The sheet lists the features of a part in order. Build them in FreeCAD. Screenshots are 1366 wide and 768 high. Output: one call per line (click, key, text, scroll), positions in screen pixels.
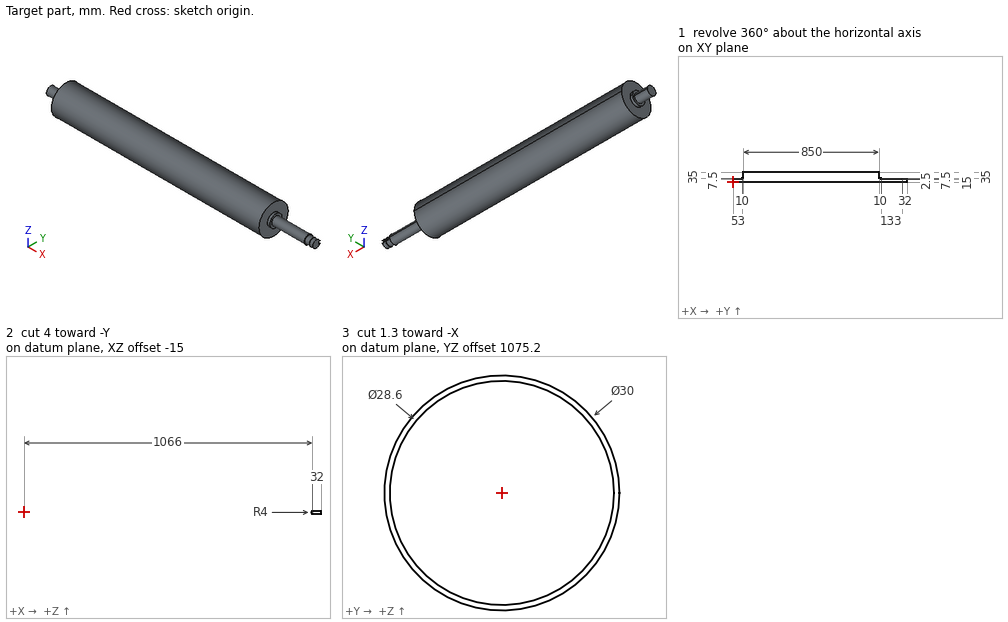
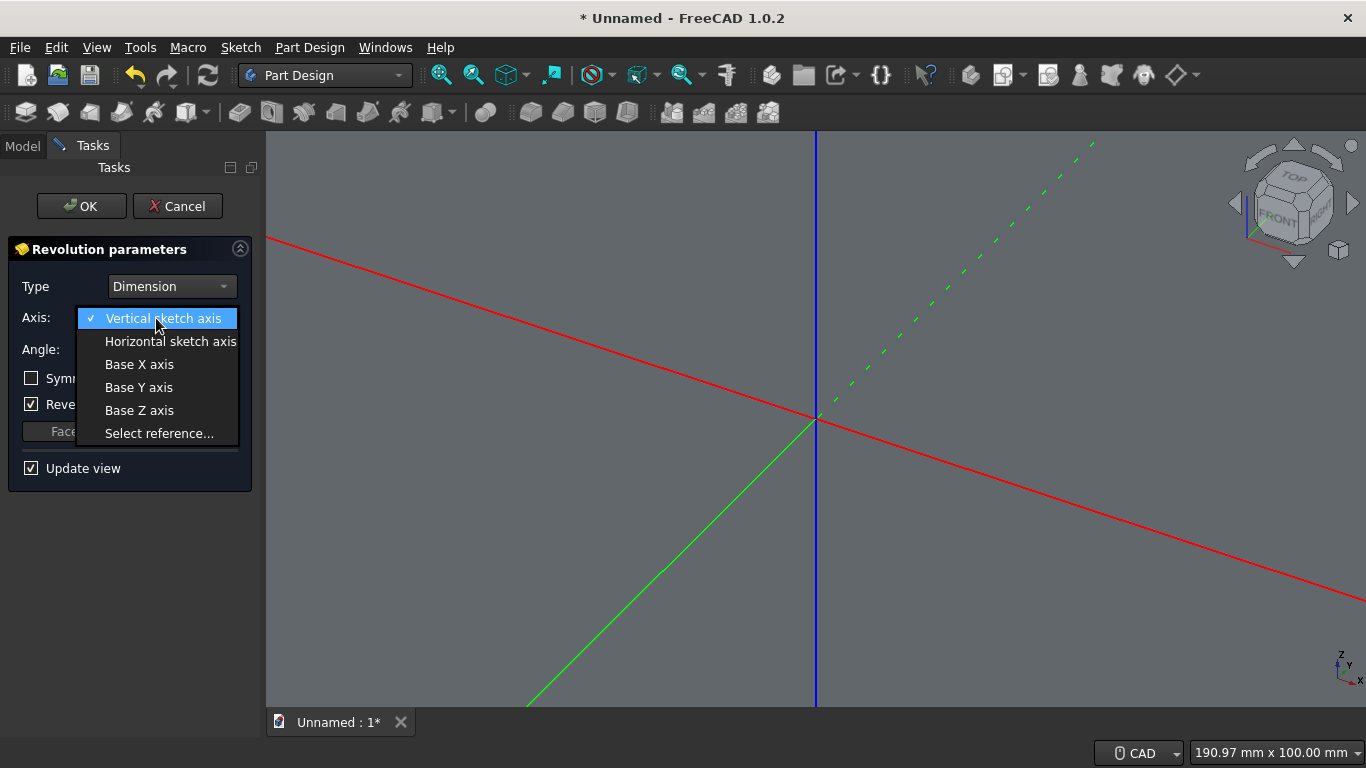
click(156, 342)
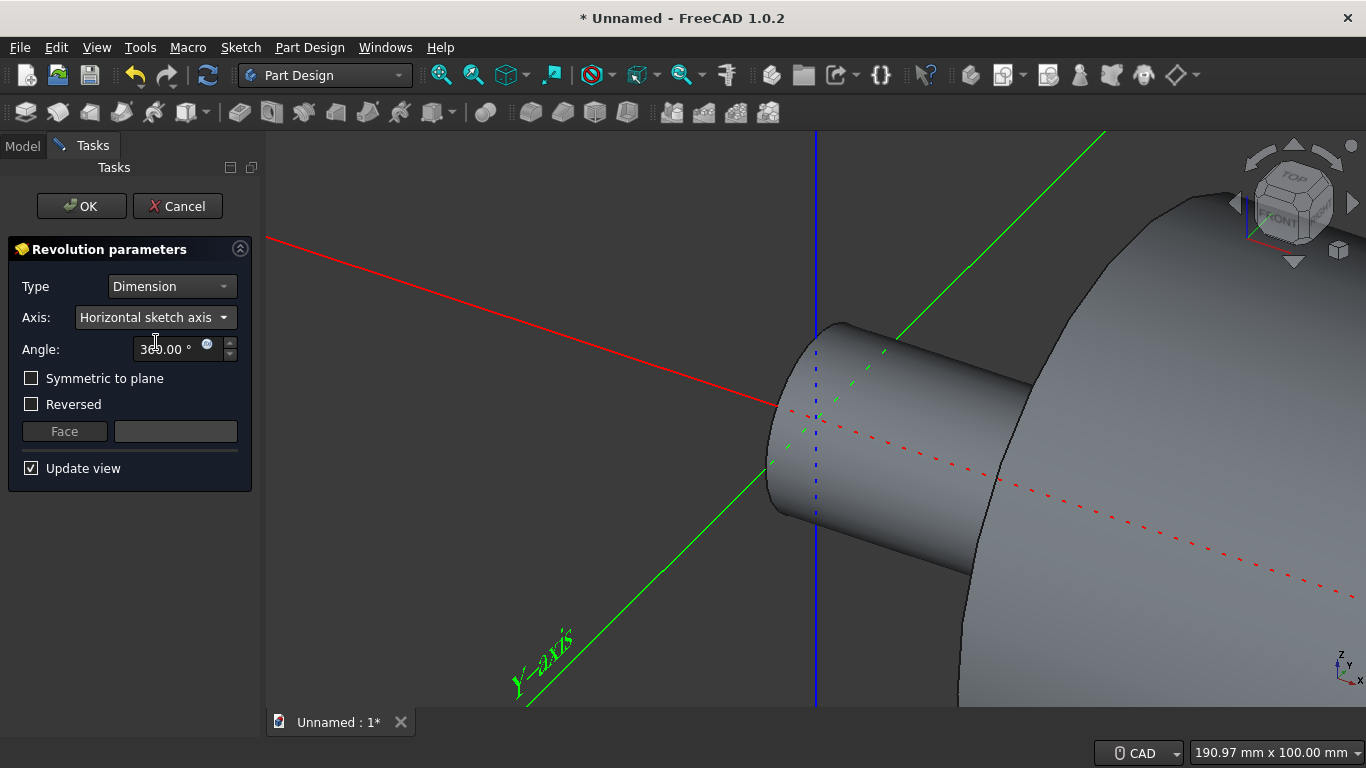
click(82, 206)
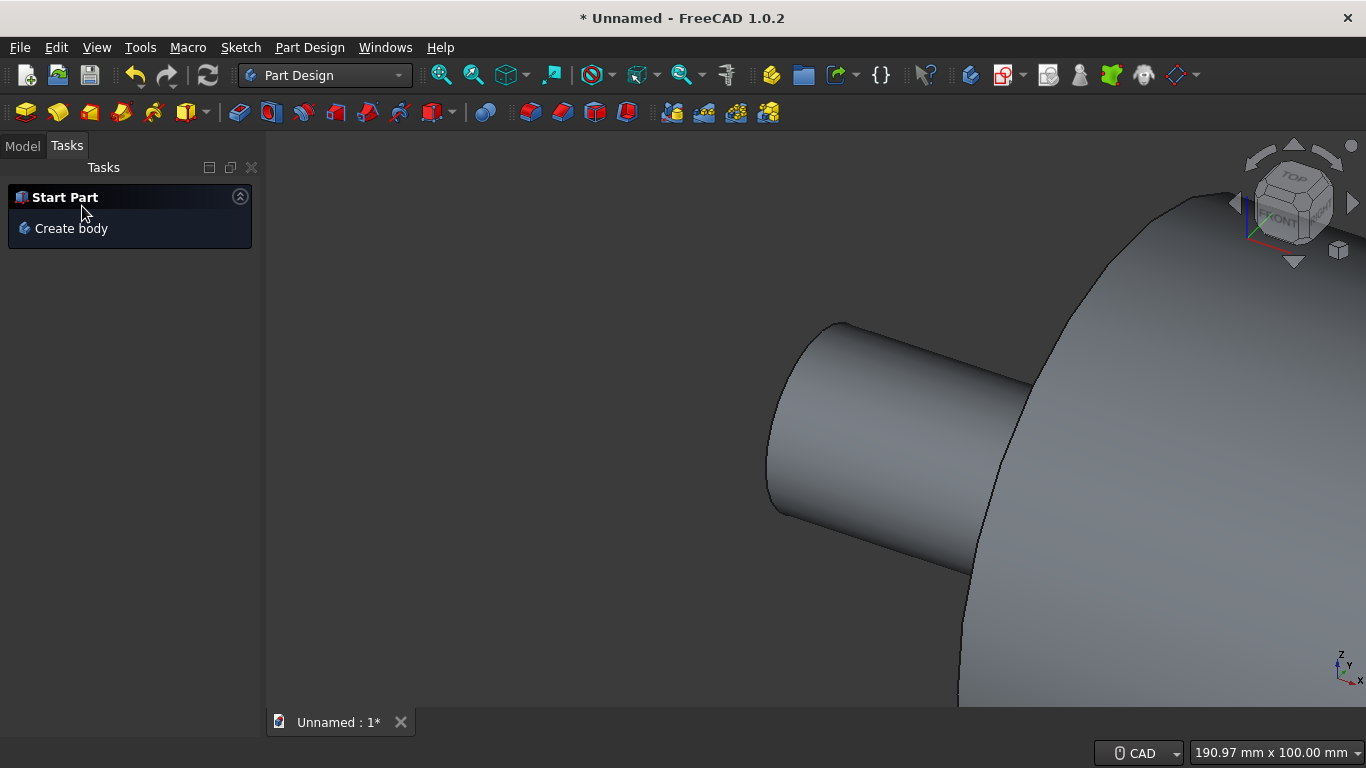
click(442, 76)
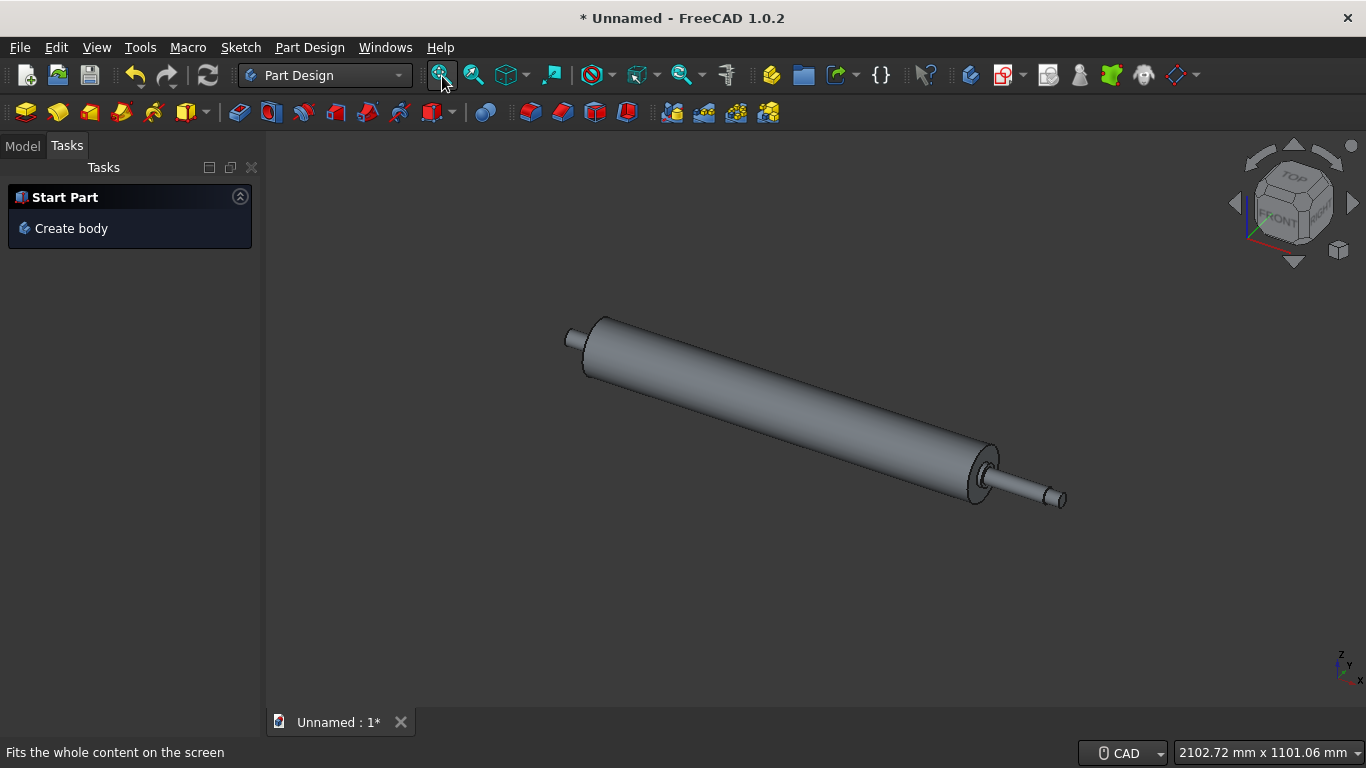
click(23, 145)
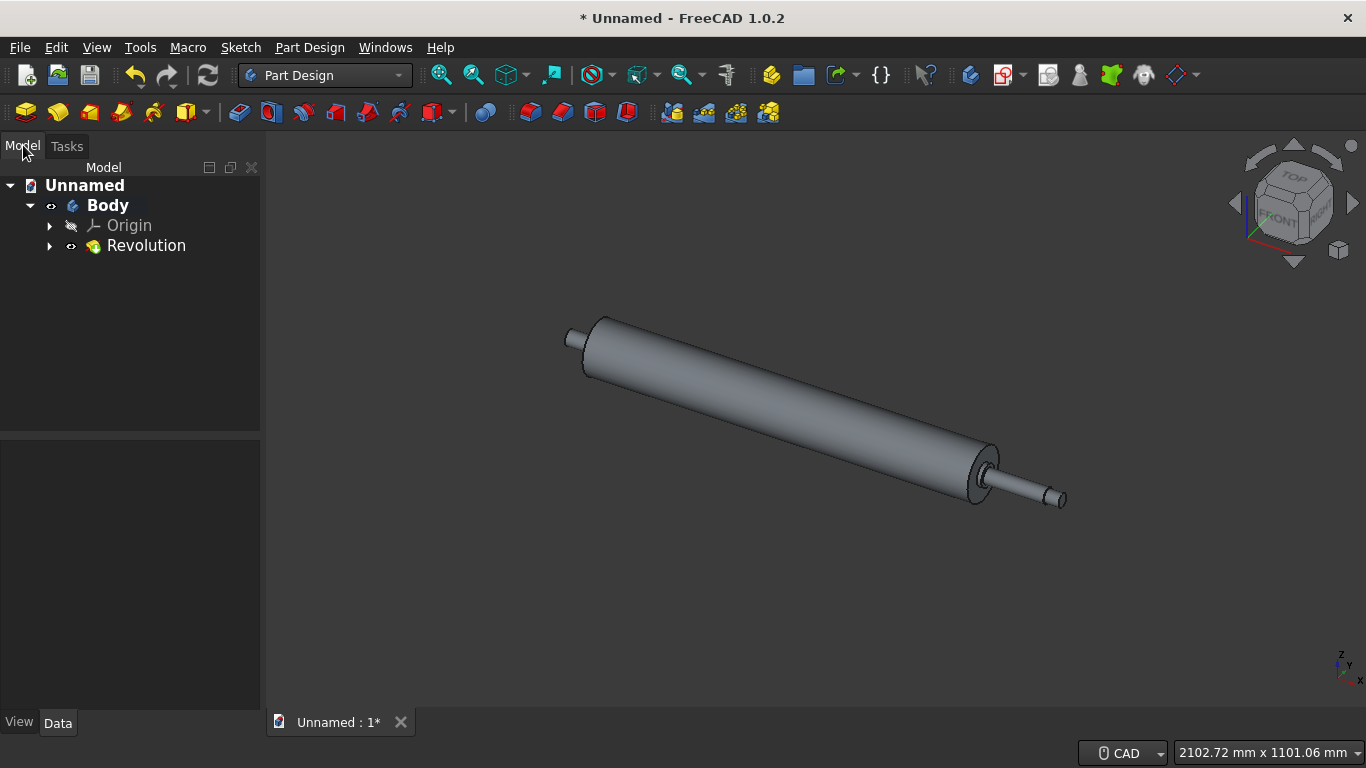
click(50, 226)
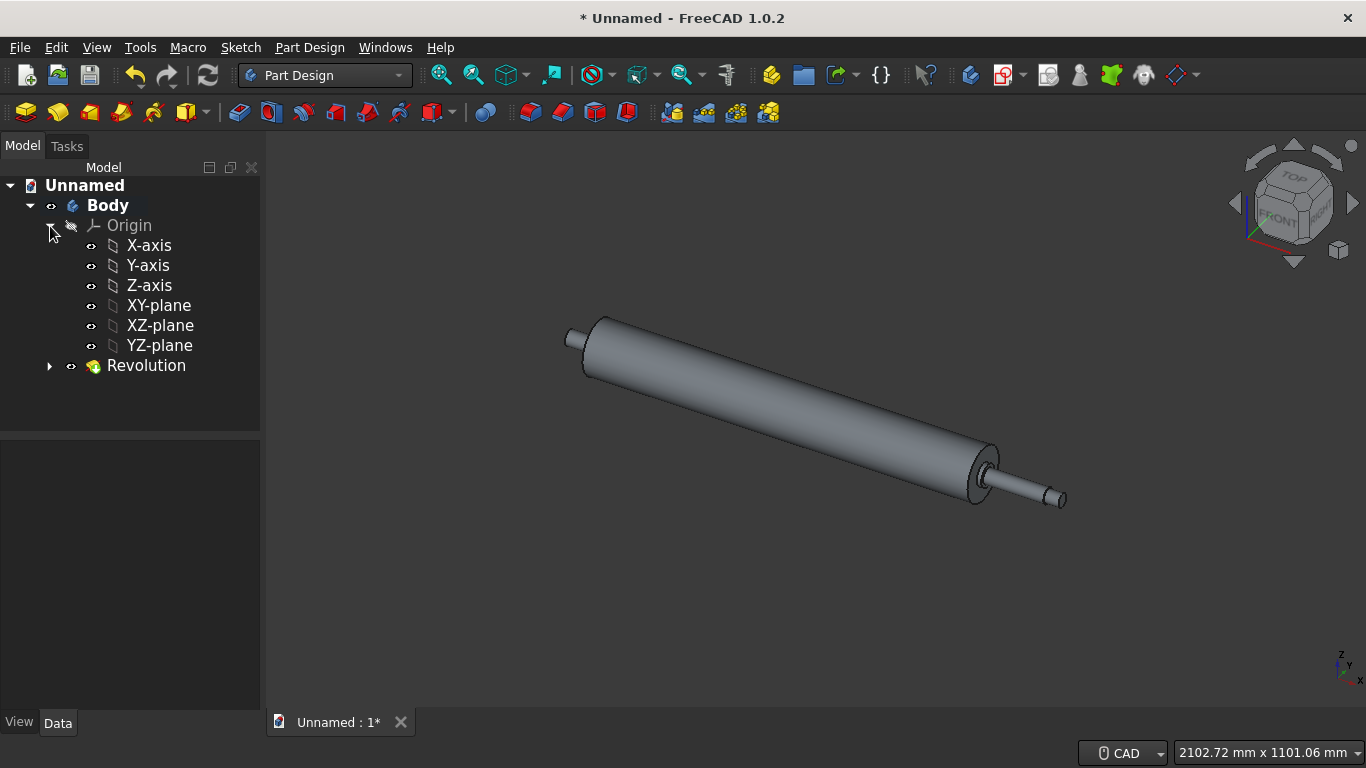
click(136, 326)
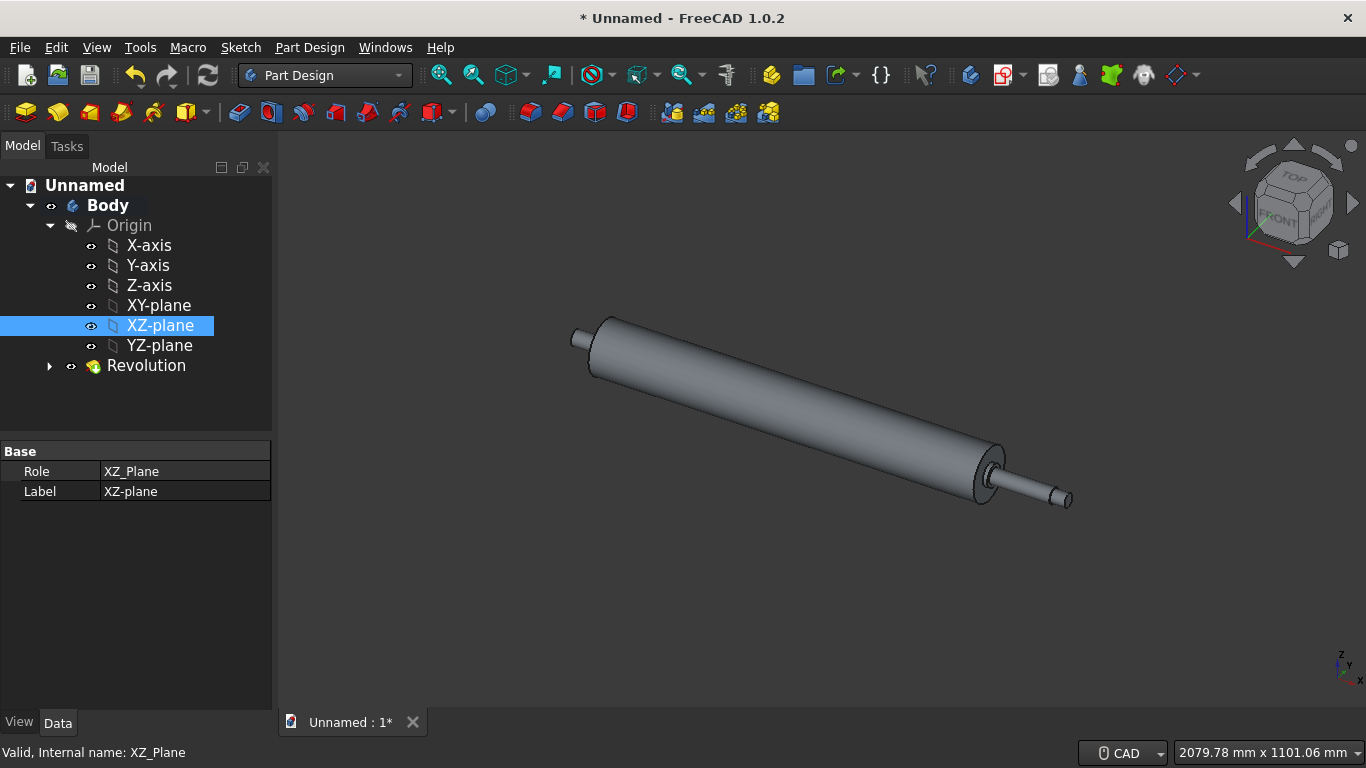
click(1176, 76)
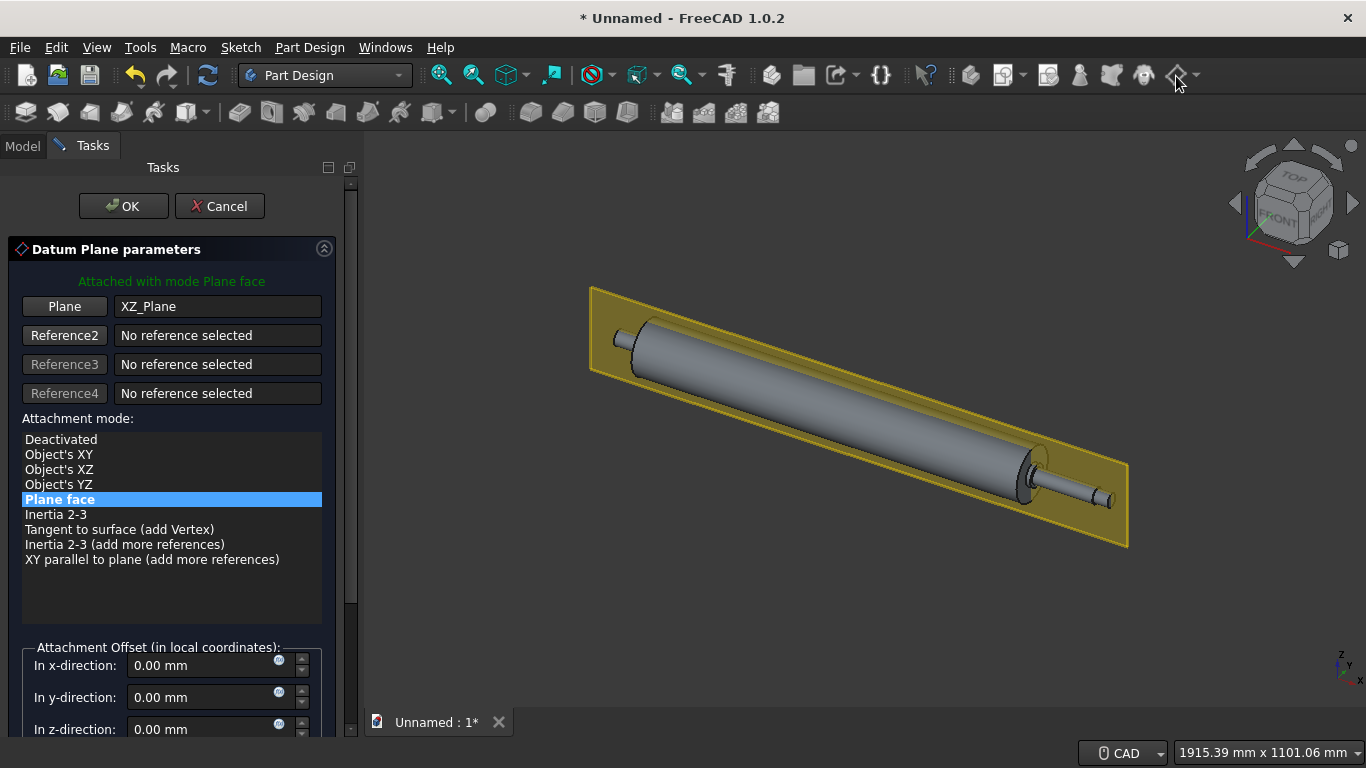
scroll(351, 456, down, 2)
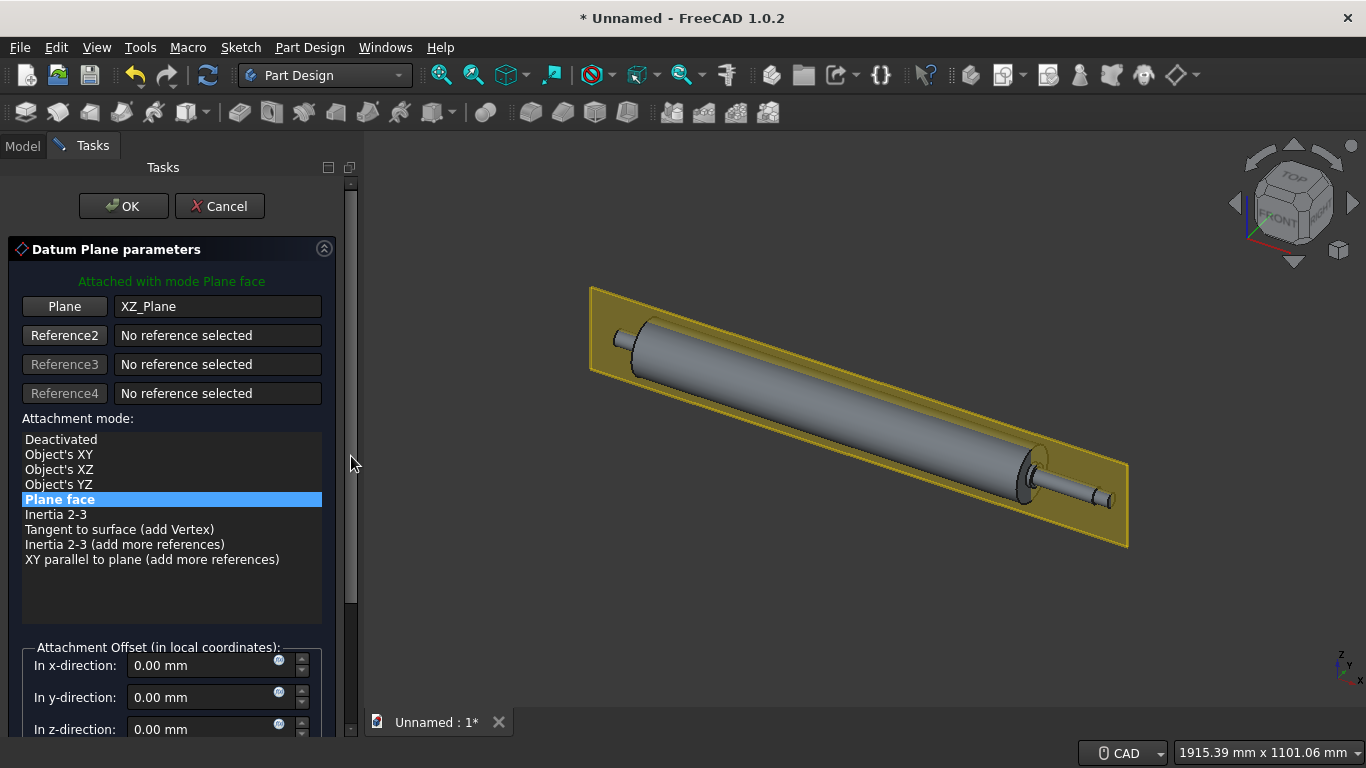
triple_click(210, 609)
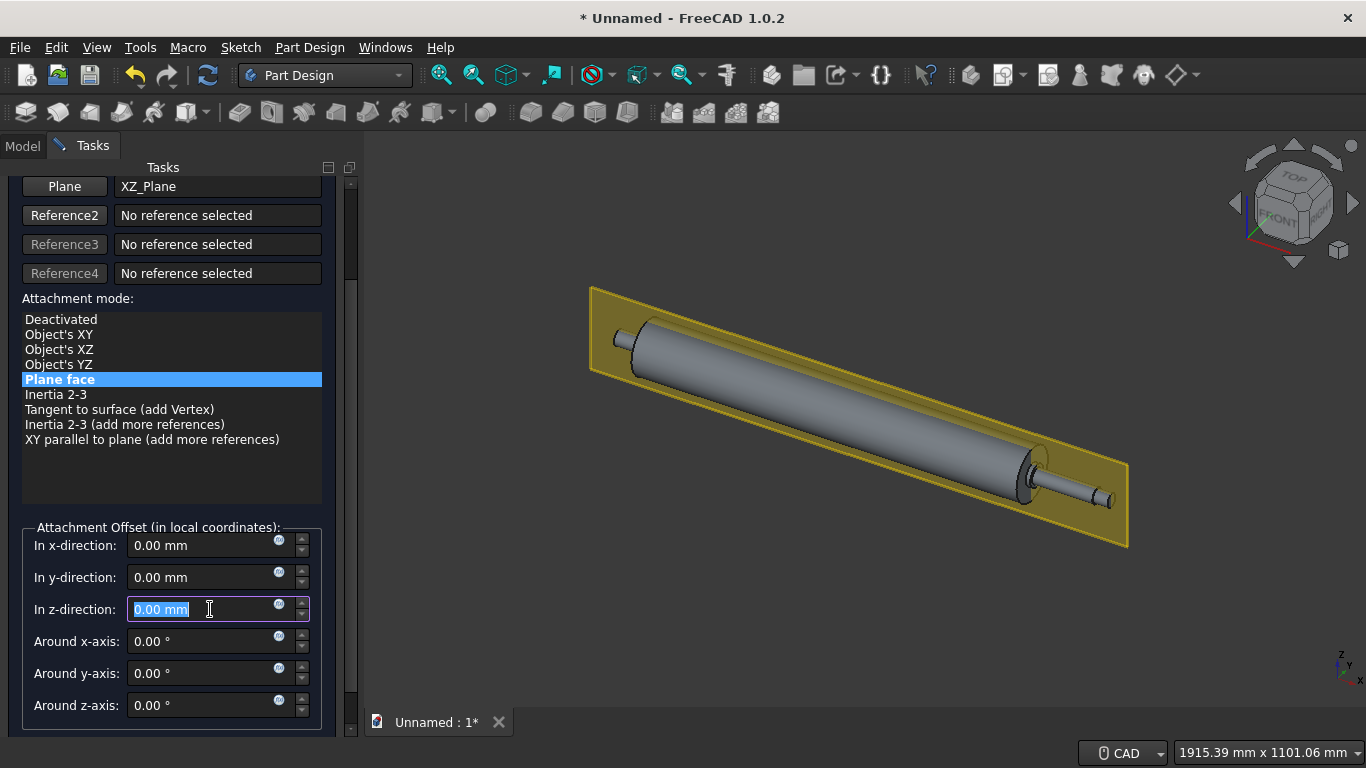
text(-15)
key(Tab)